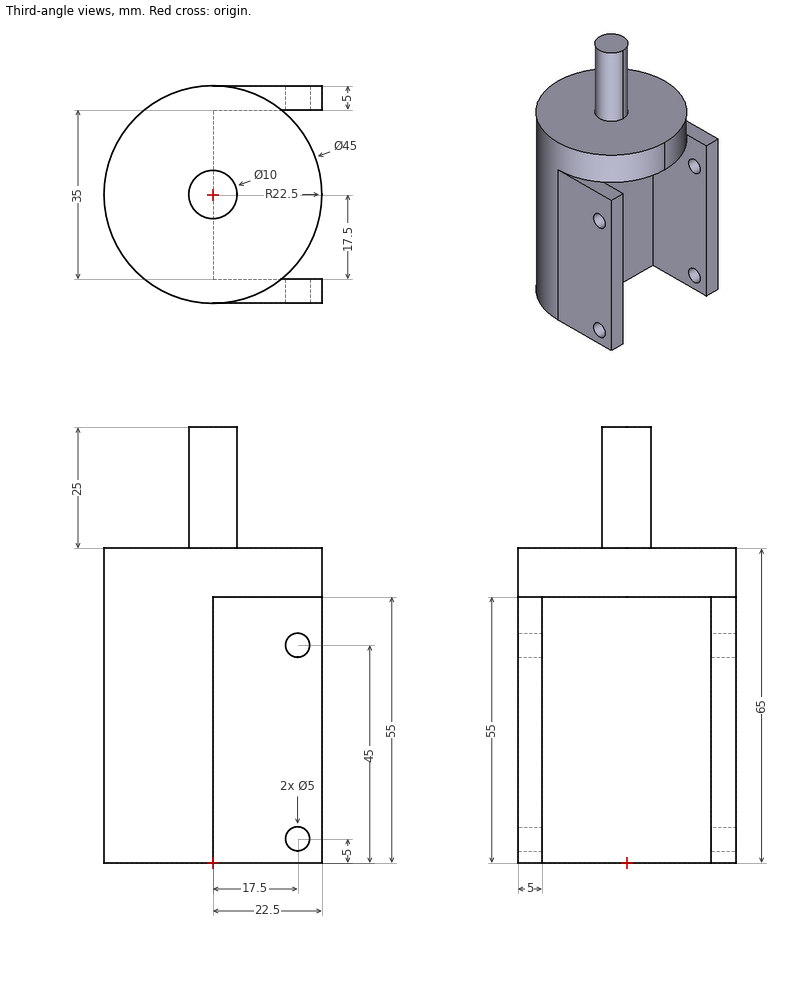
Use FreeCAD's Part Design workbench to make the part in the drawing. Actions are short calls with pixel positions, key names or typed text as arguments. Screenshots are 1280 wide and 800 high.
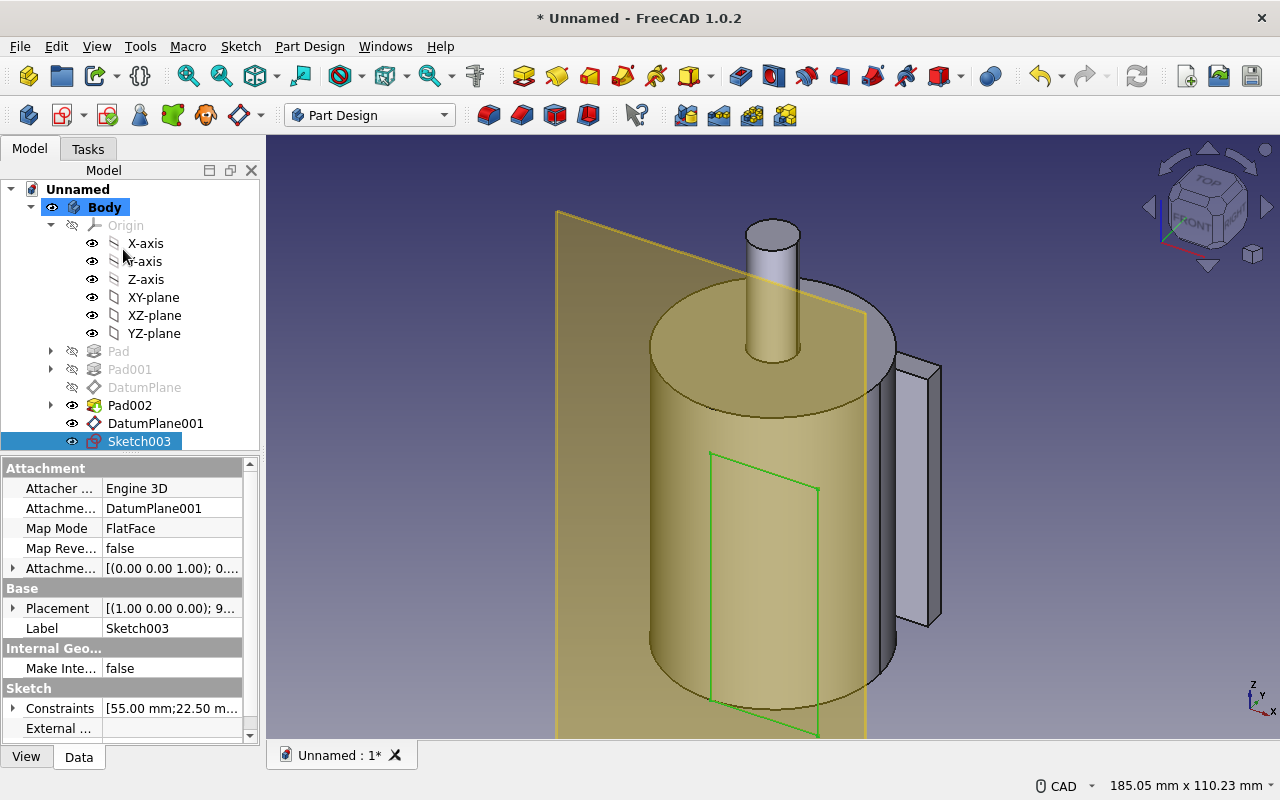
click(524, 76)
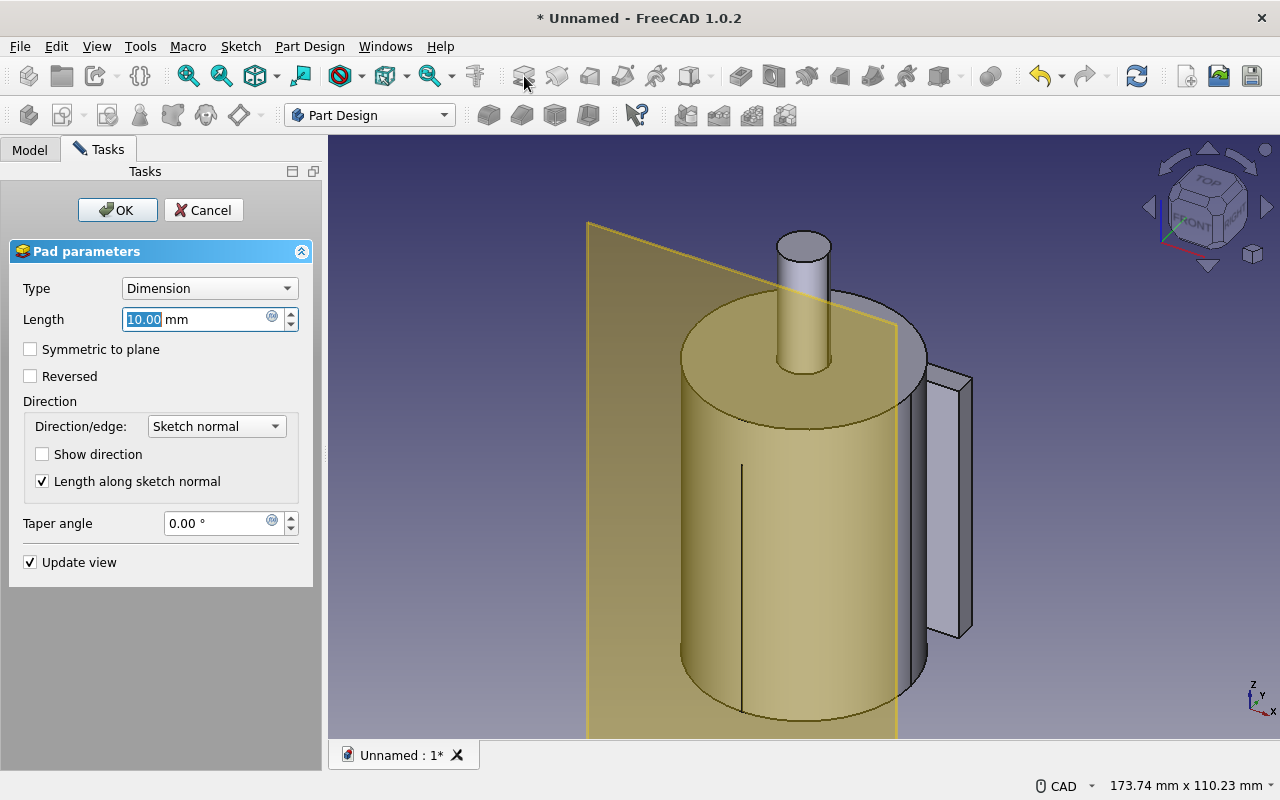
text(5)
key(Tab)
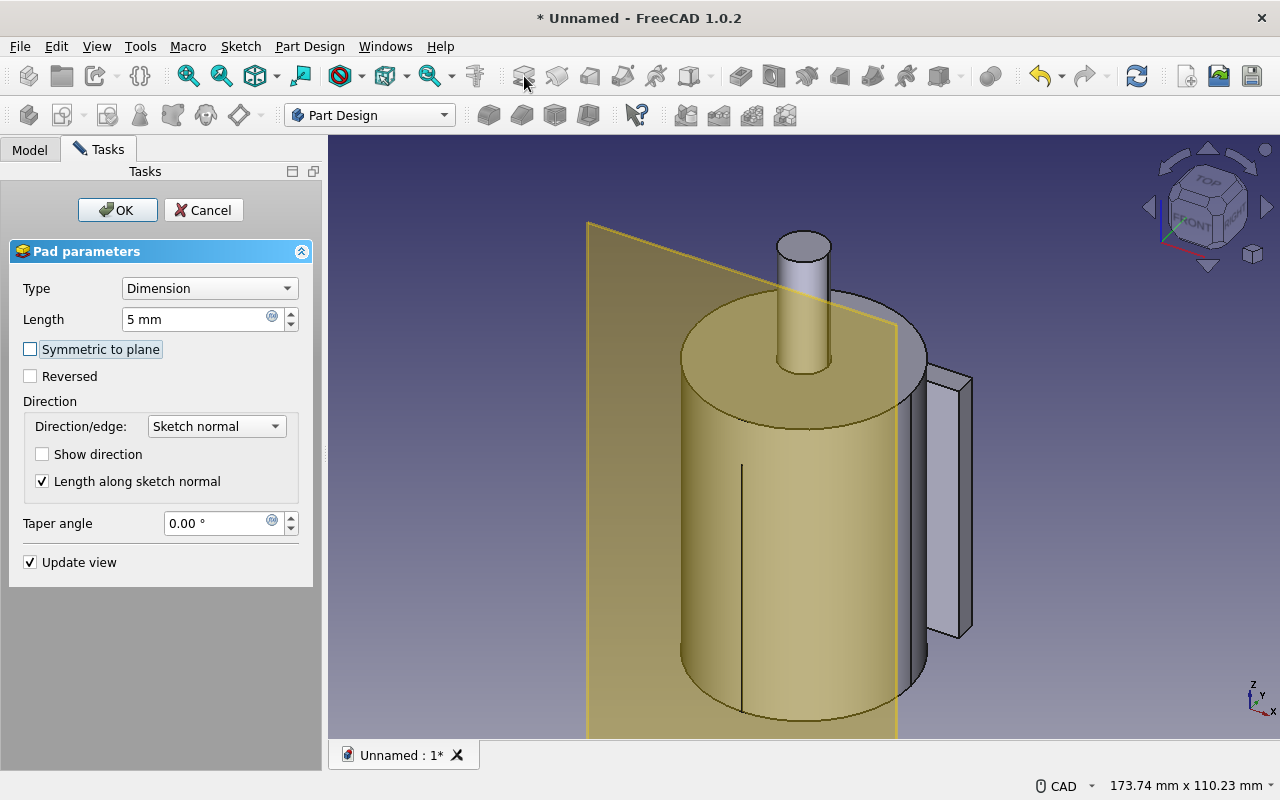
click(31, 376)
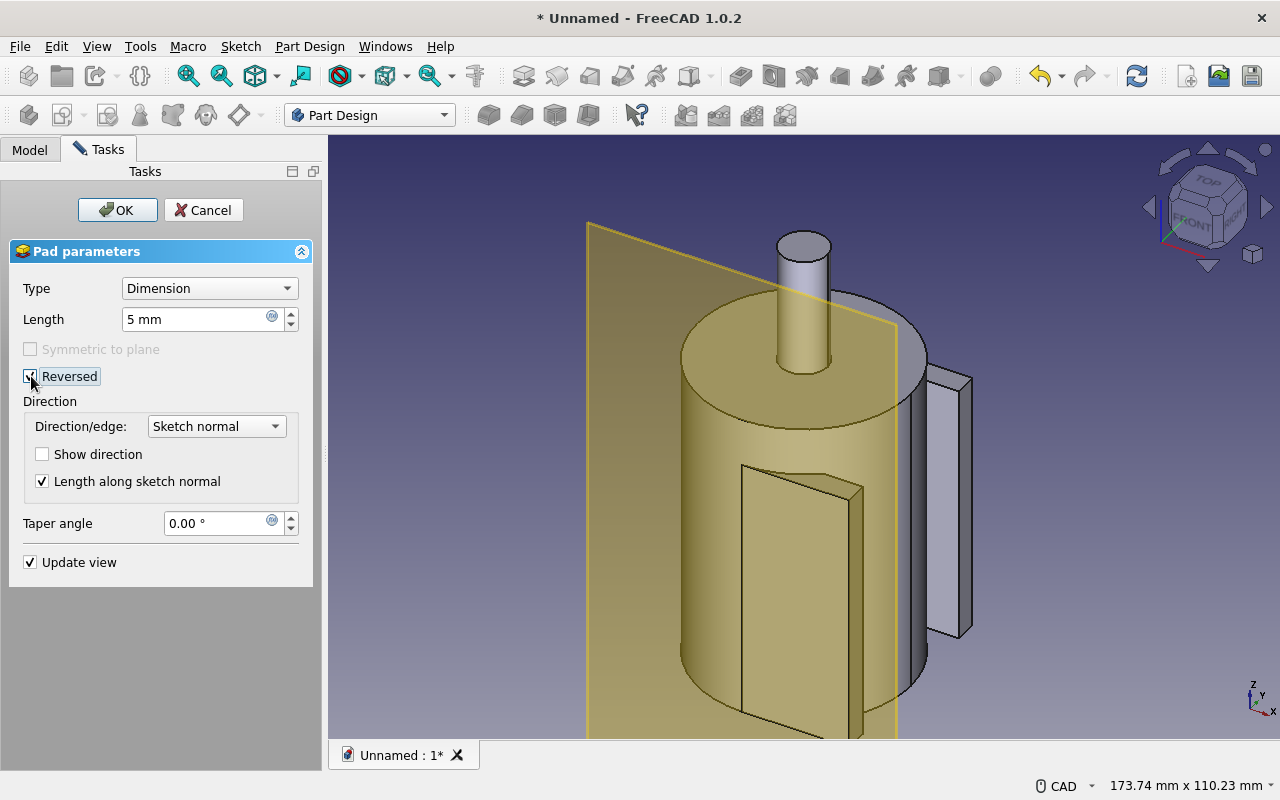
click(118, 210)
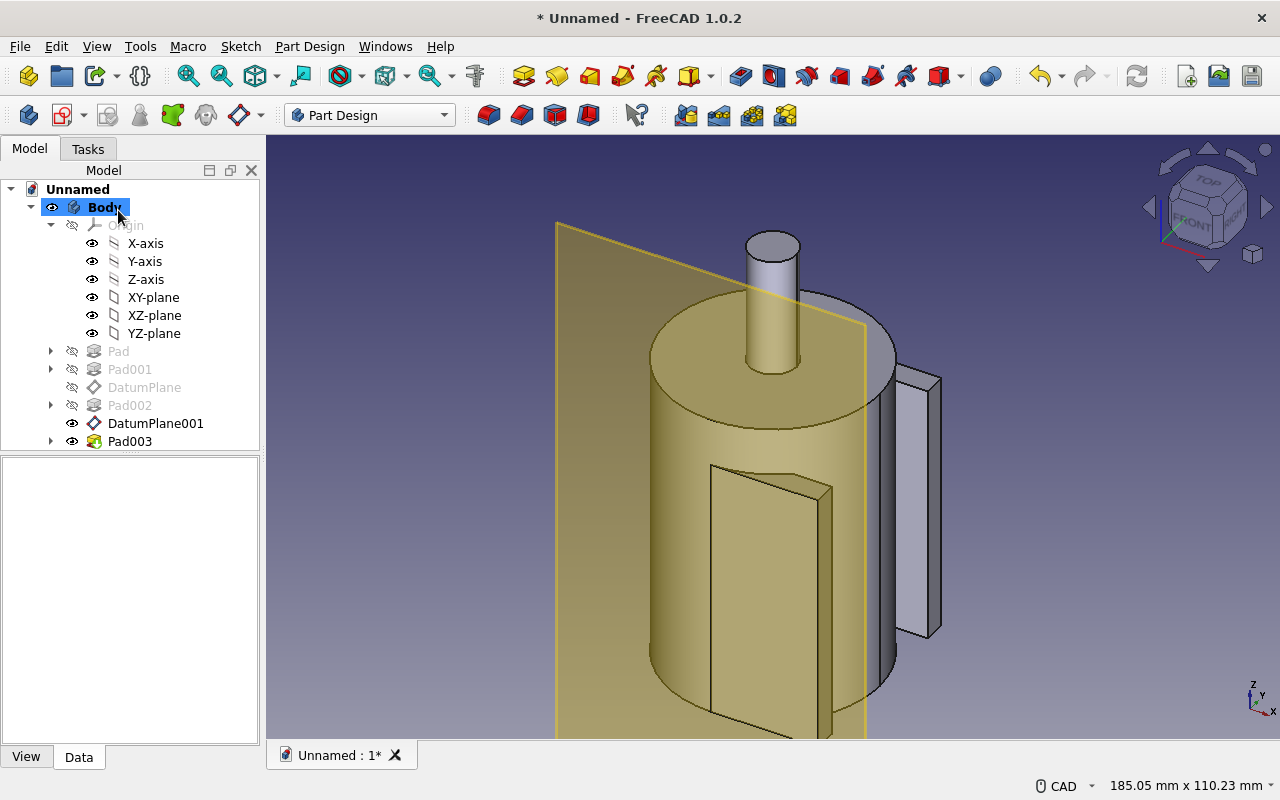
click(117, 423)
key(space)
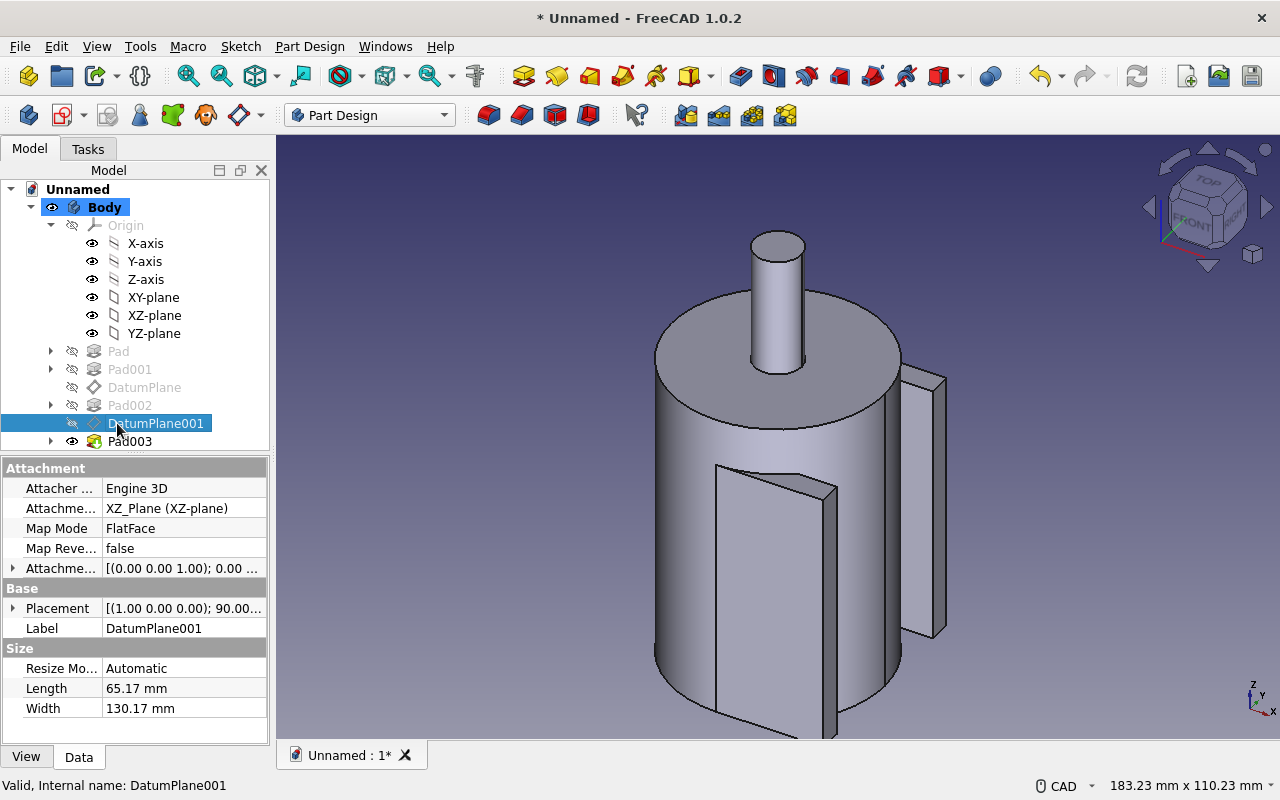
click(189, 76)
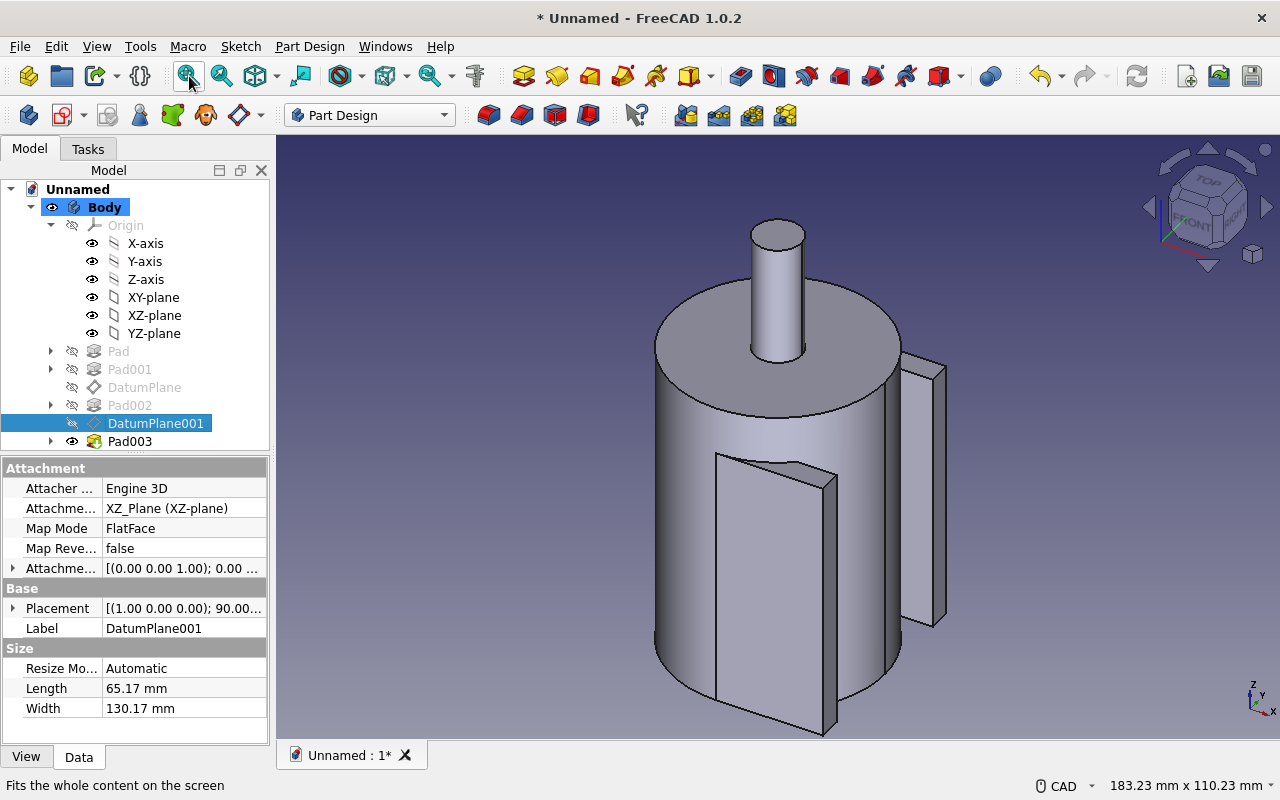
key(5)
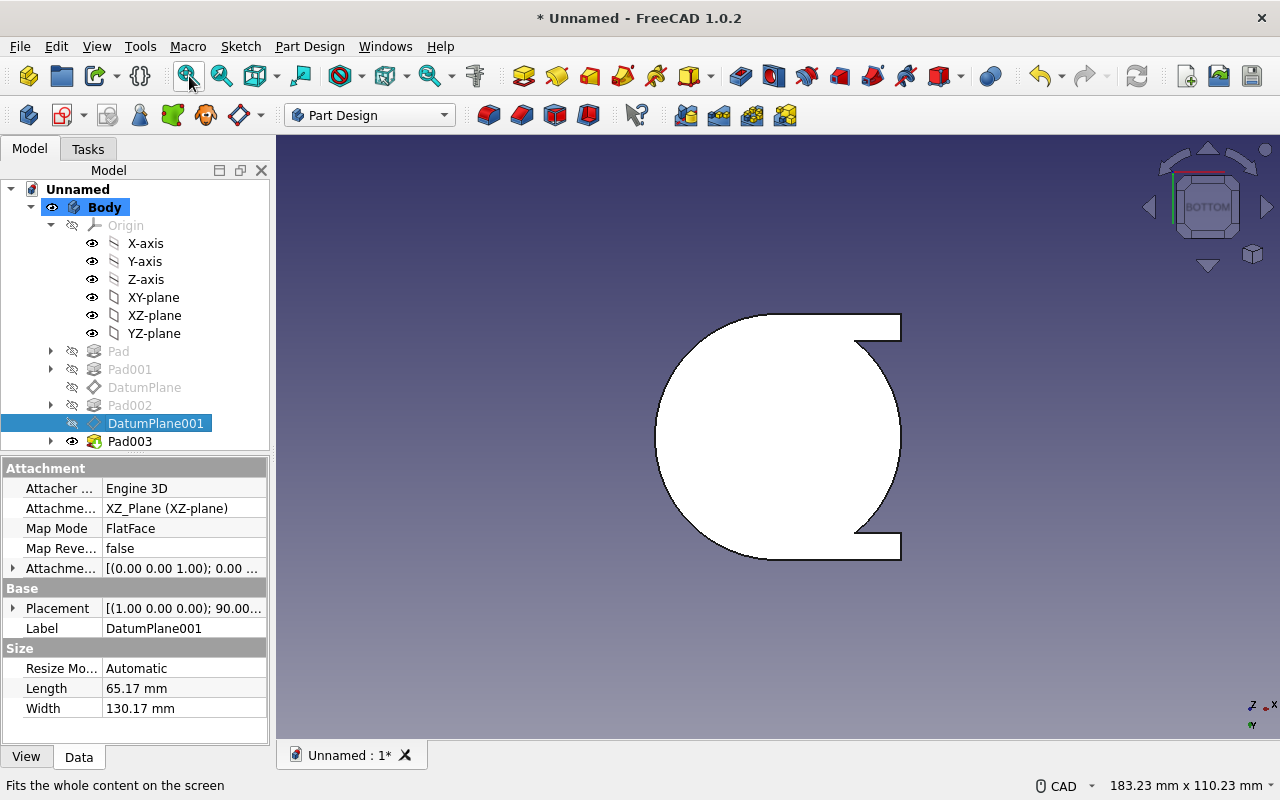
click(189, 76)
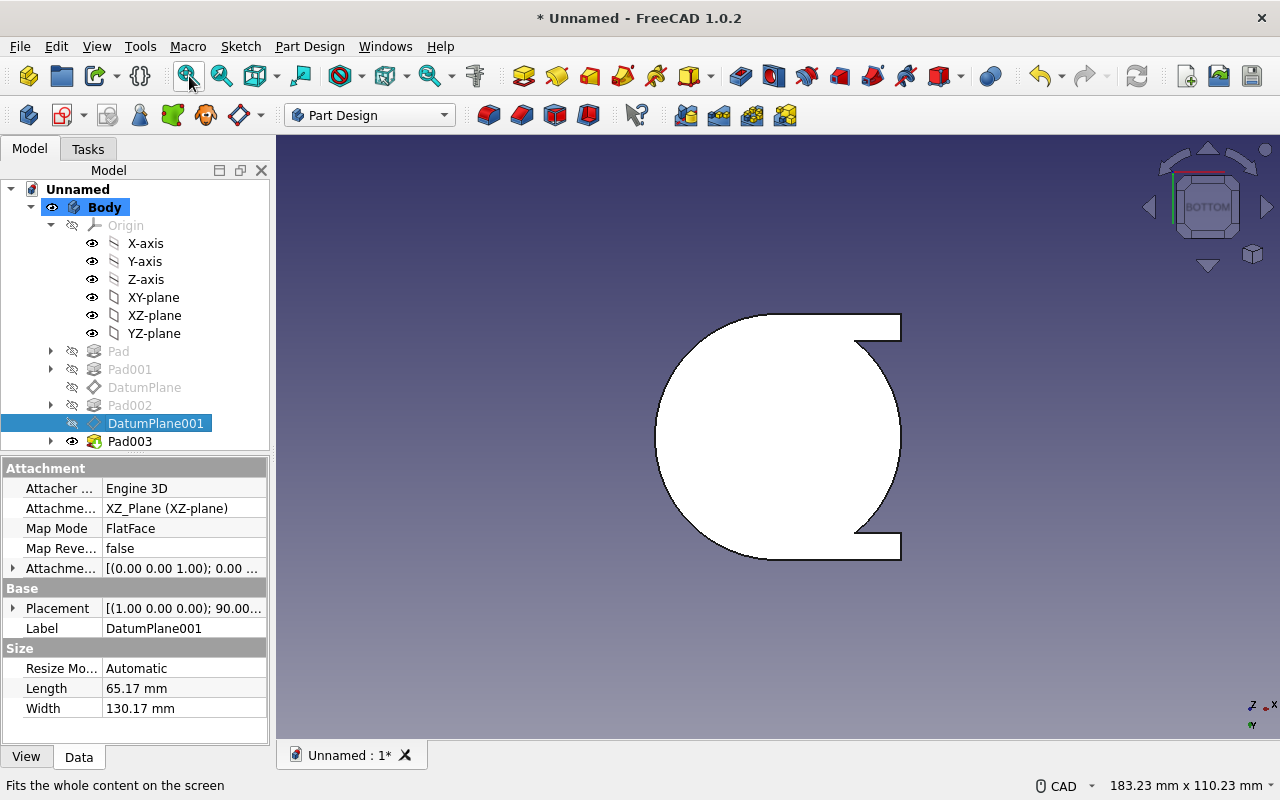
click(778, 436)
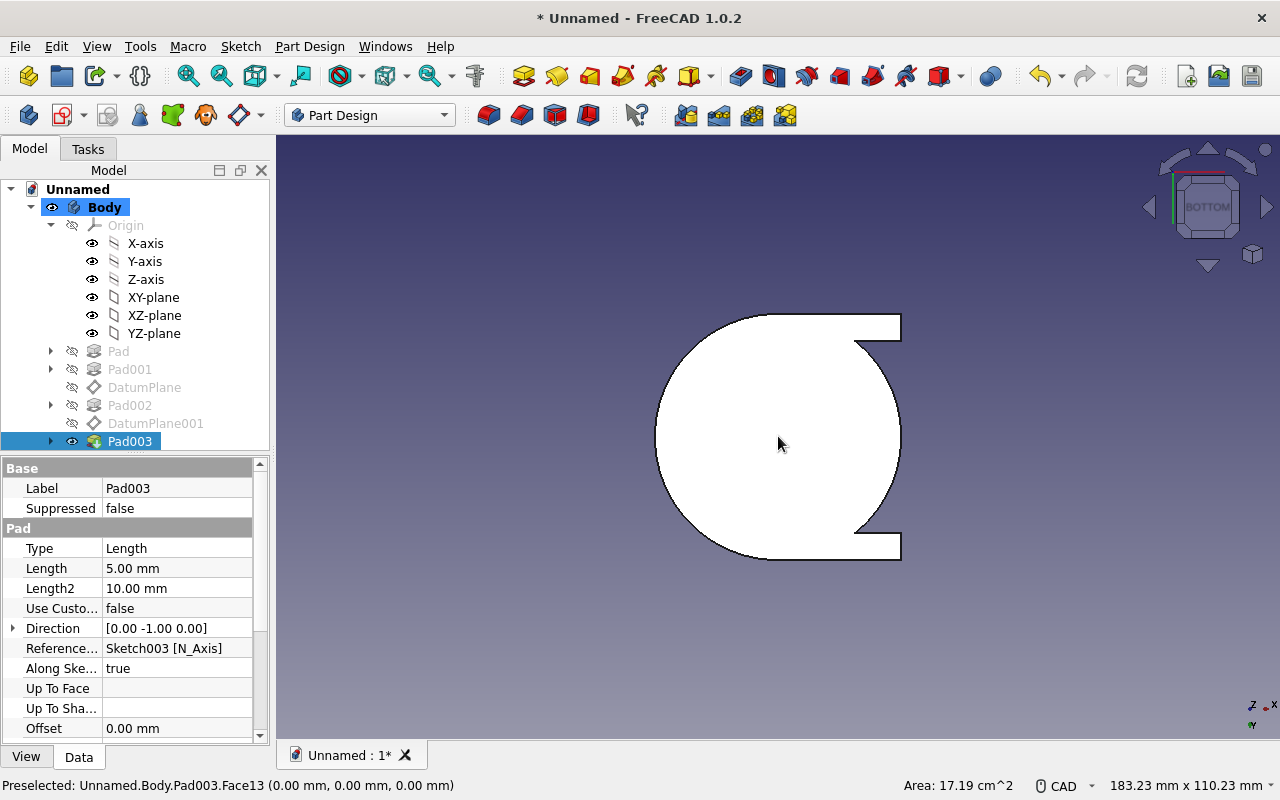
click(62, 116)